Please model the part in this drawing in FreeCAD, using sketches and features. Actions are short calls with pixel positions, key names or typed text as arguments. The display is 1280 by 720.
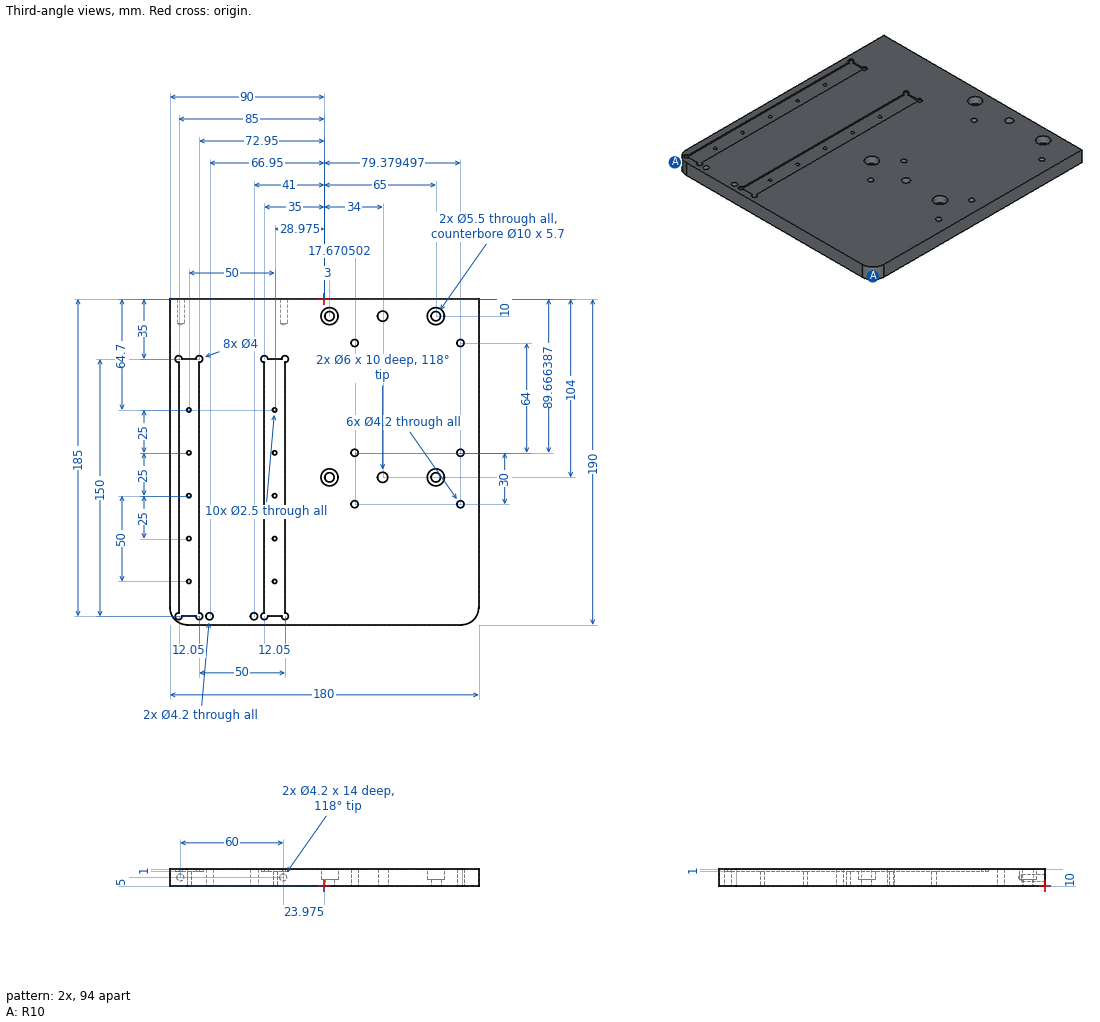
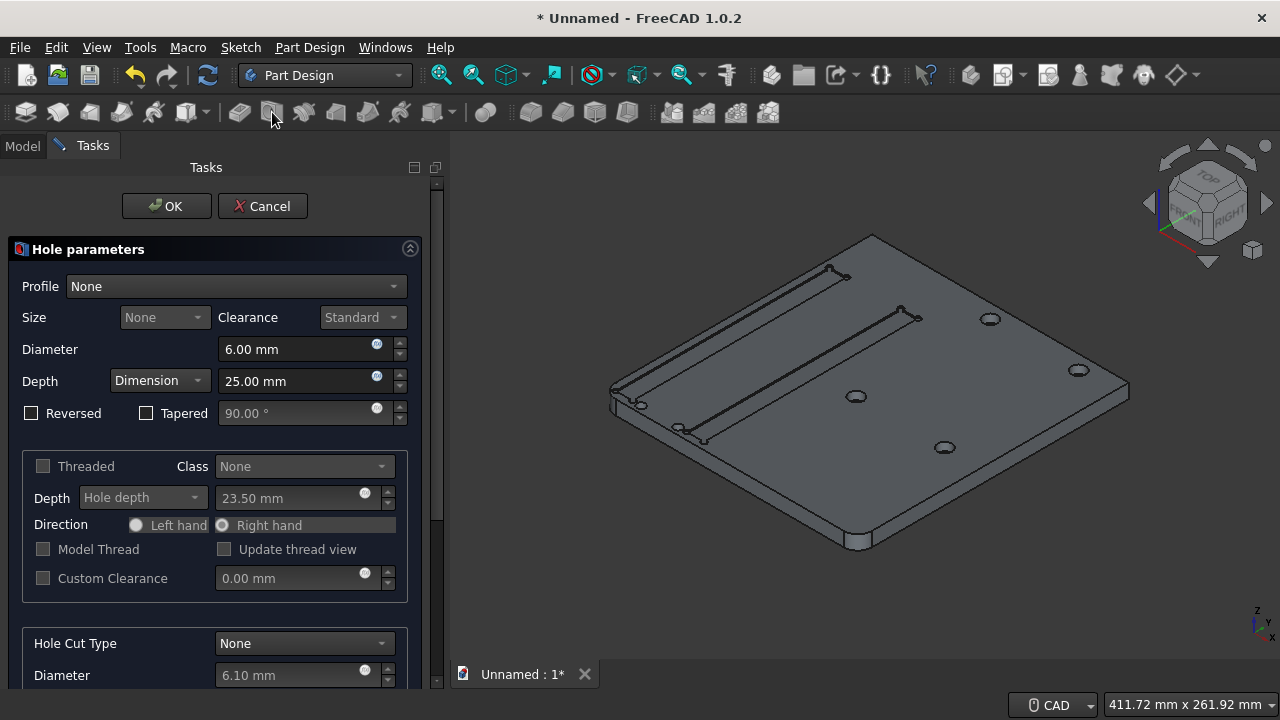
triple_click(305, 349)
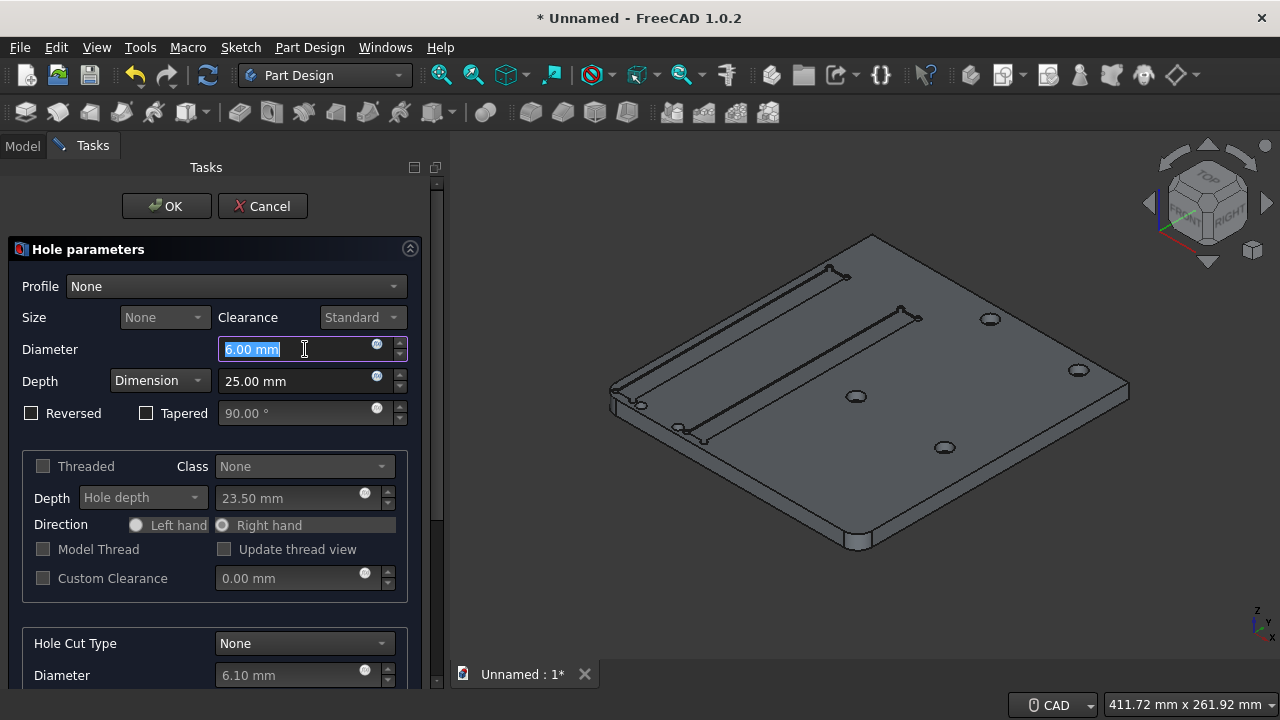
text(4.2)
key(Tab)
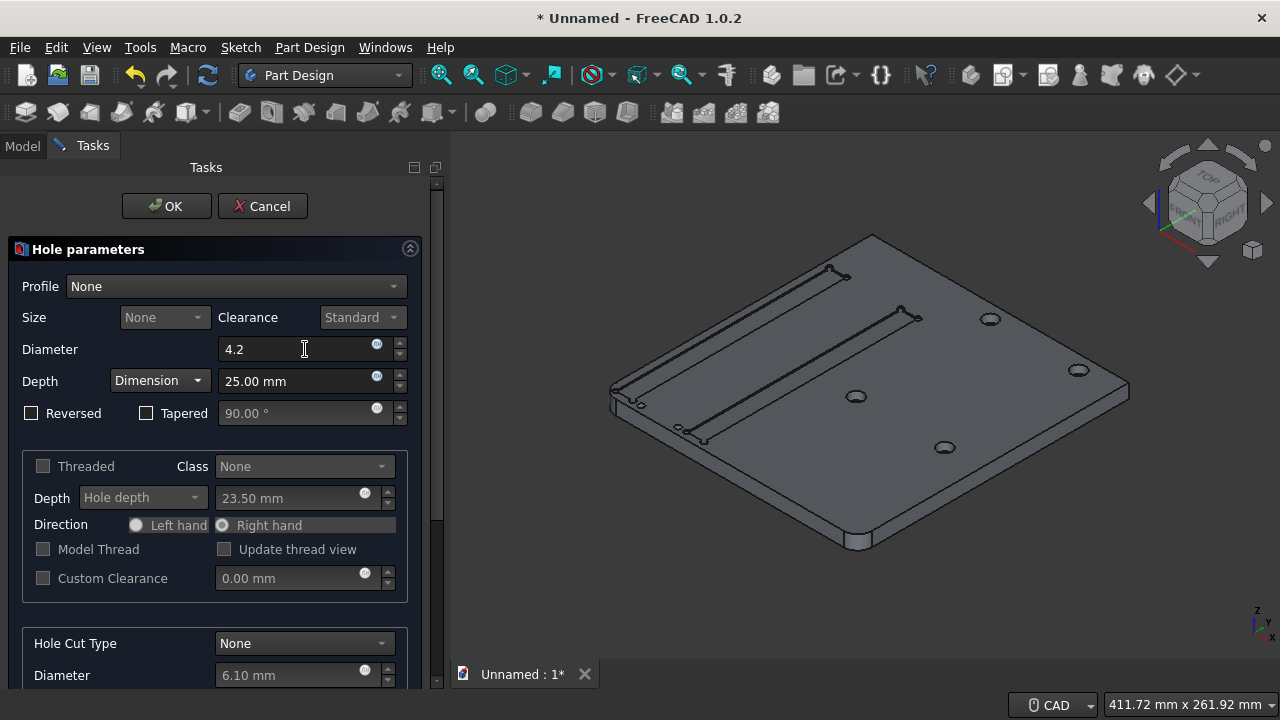
click(161, 380)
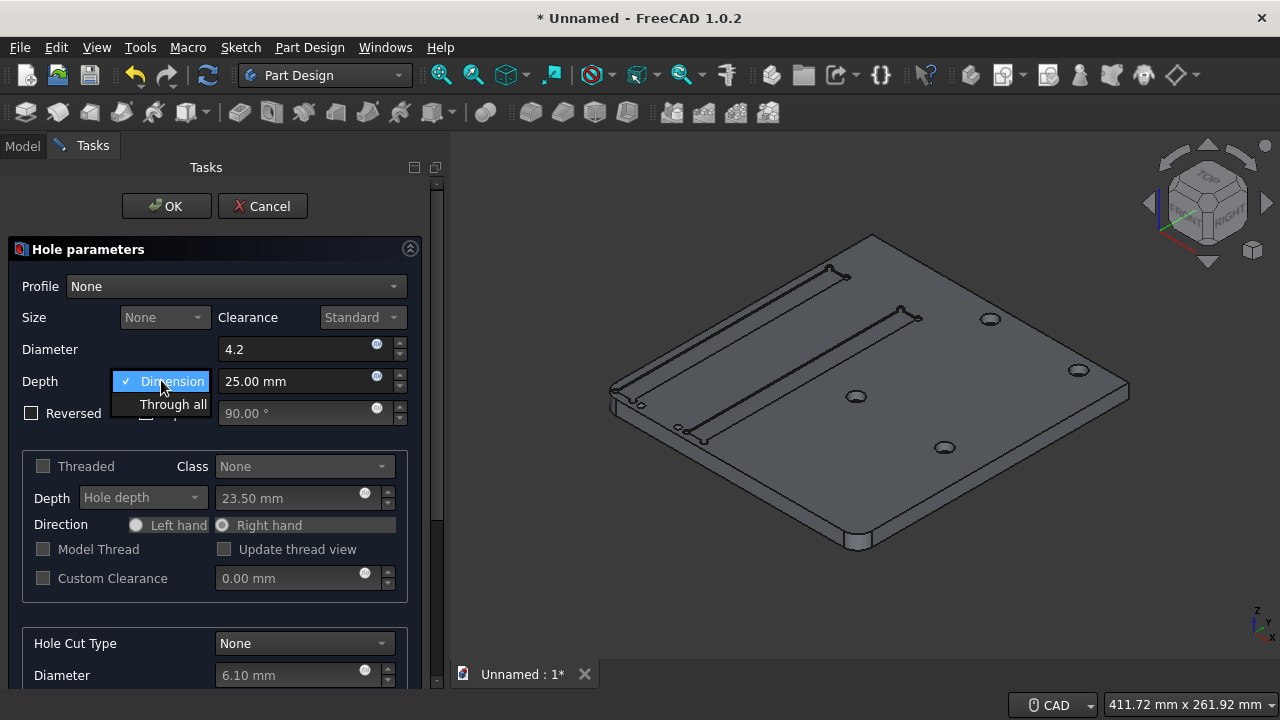
click(160, 404)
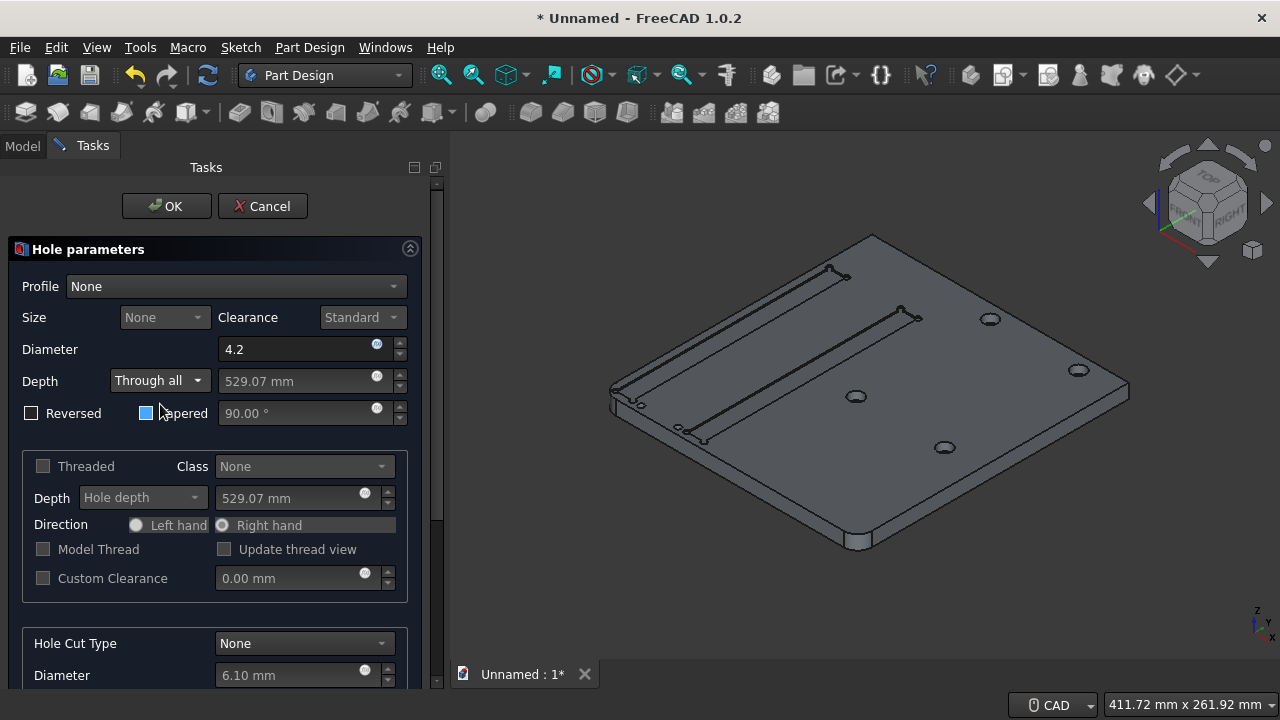
click(167, 206)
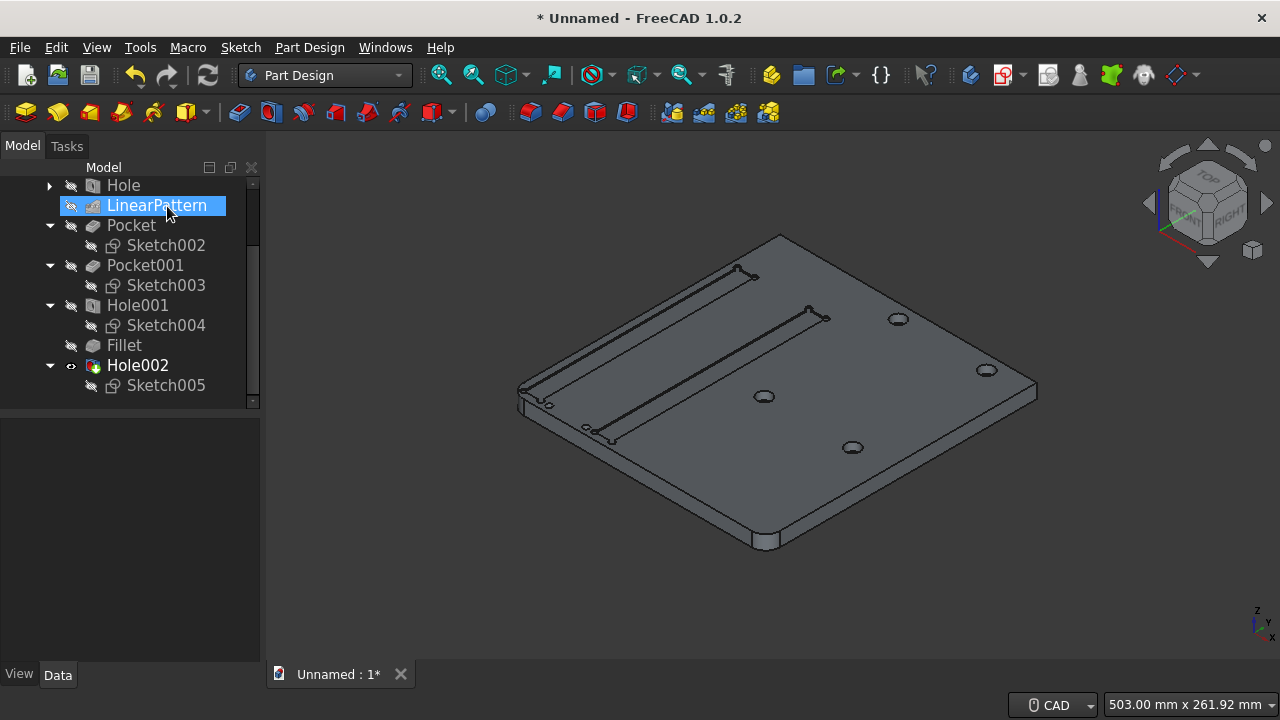
click(732, 452)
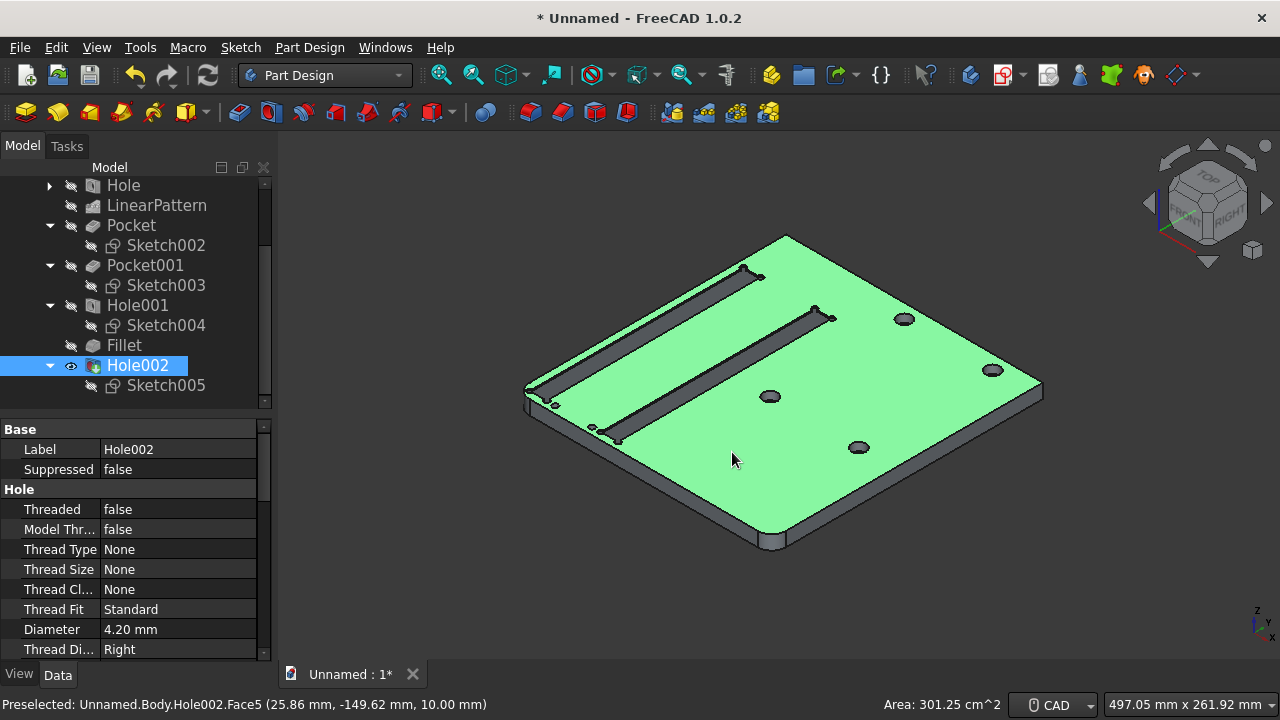
click(1004, 76)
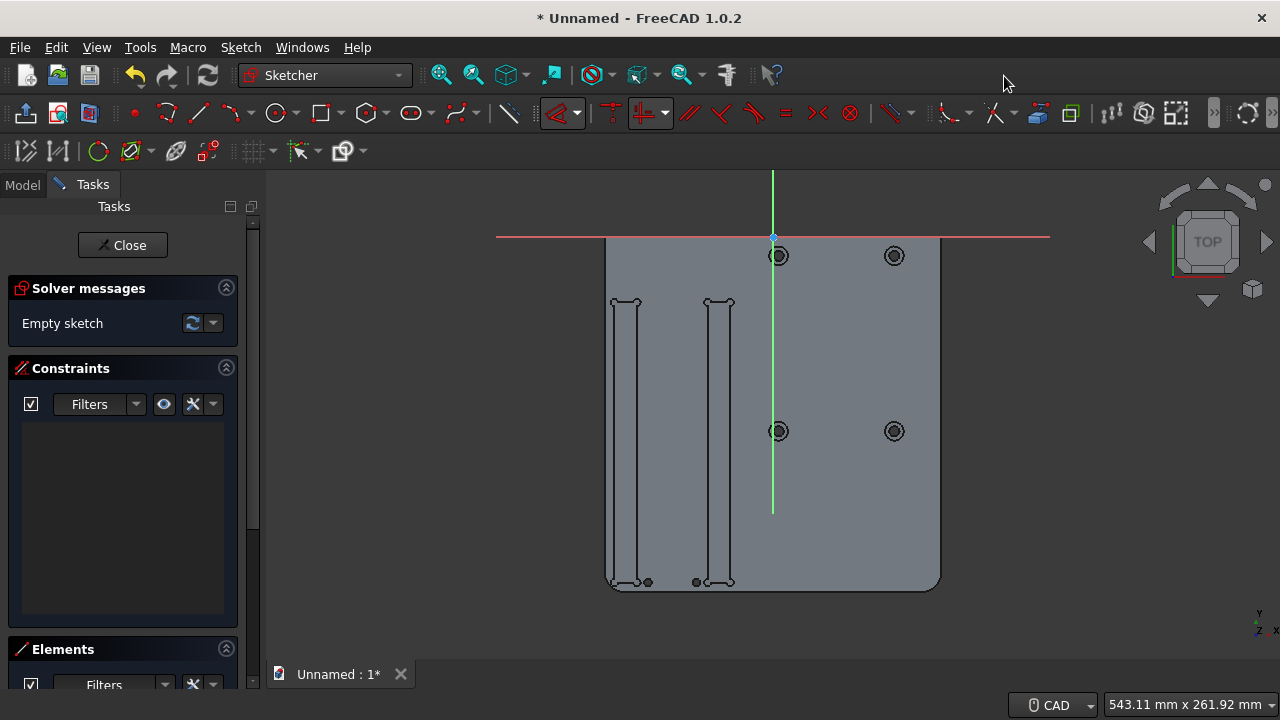
key(g)
key(c)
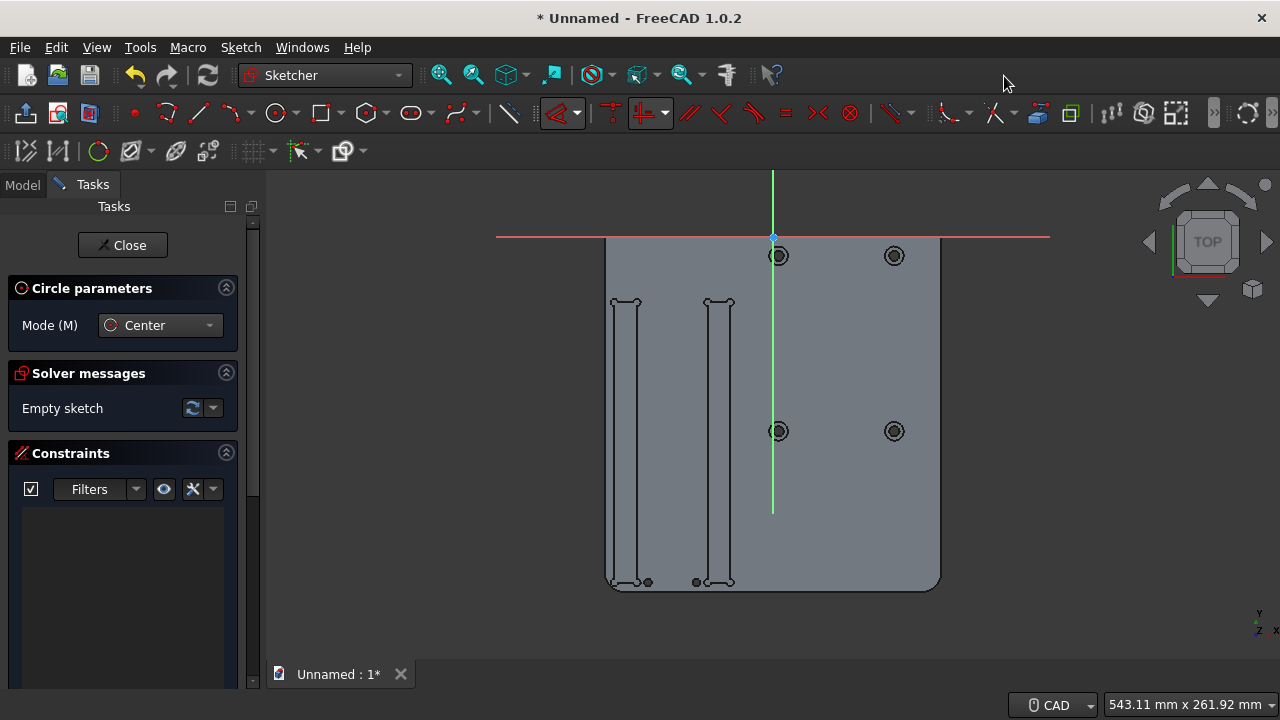
scroll(921, 461, up, 9)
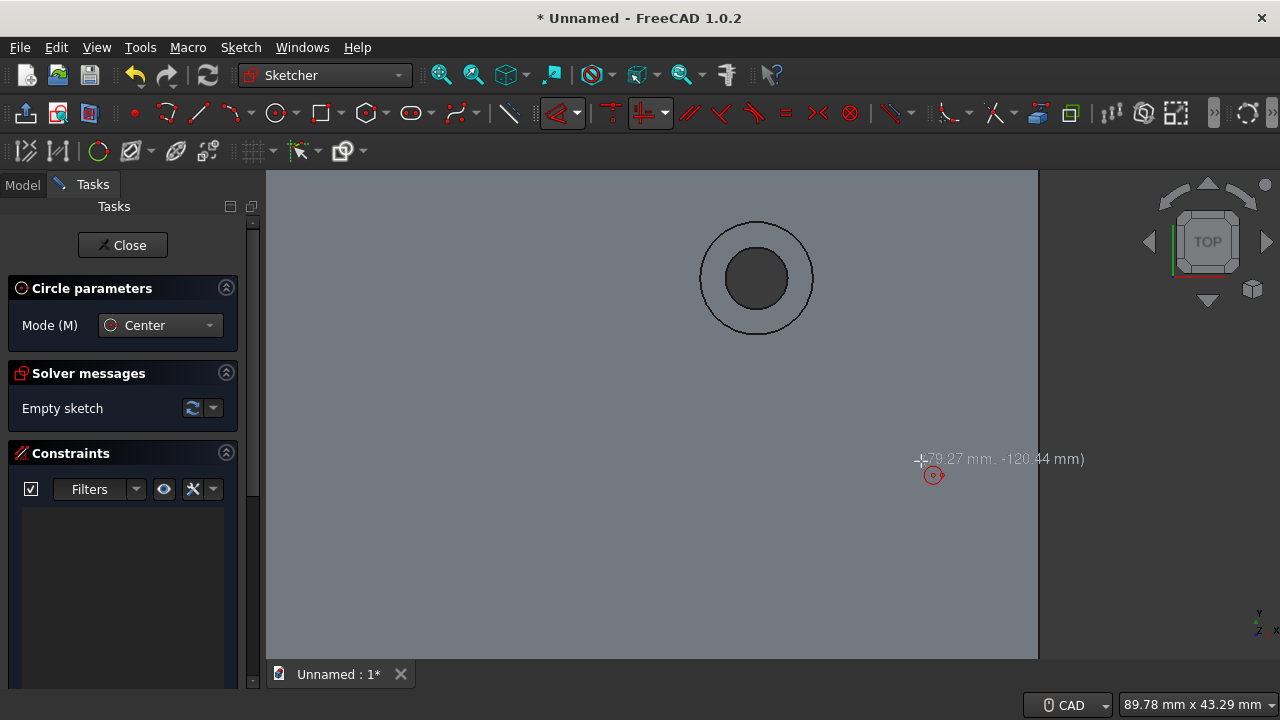
scroll(761, 572, down, 8)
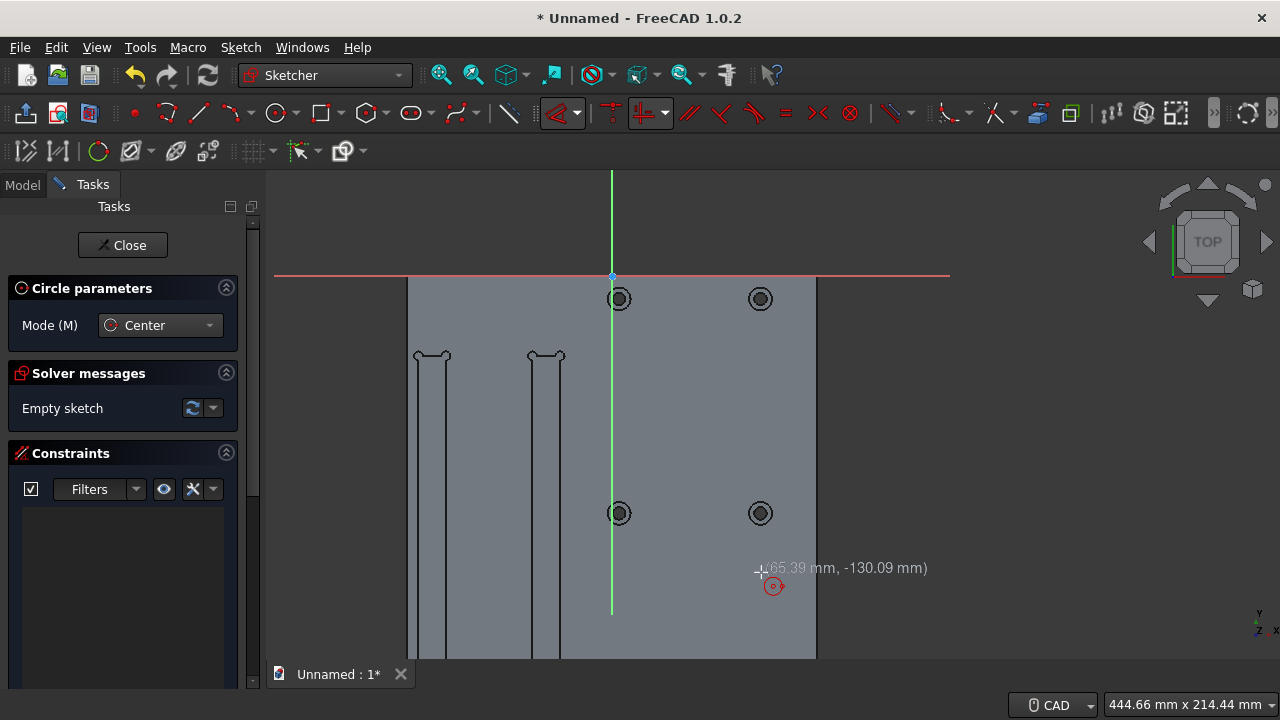
click(793, 549)
move(797, 546)